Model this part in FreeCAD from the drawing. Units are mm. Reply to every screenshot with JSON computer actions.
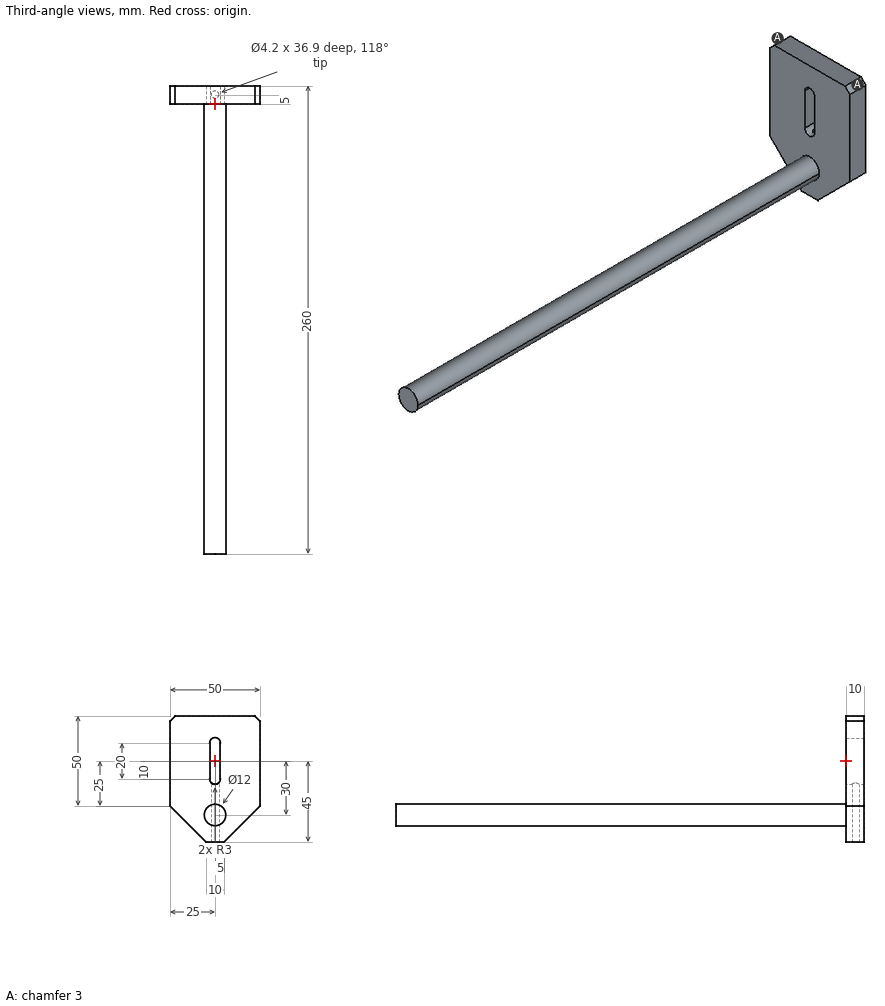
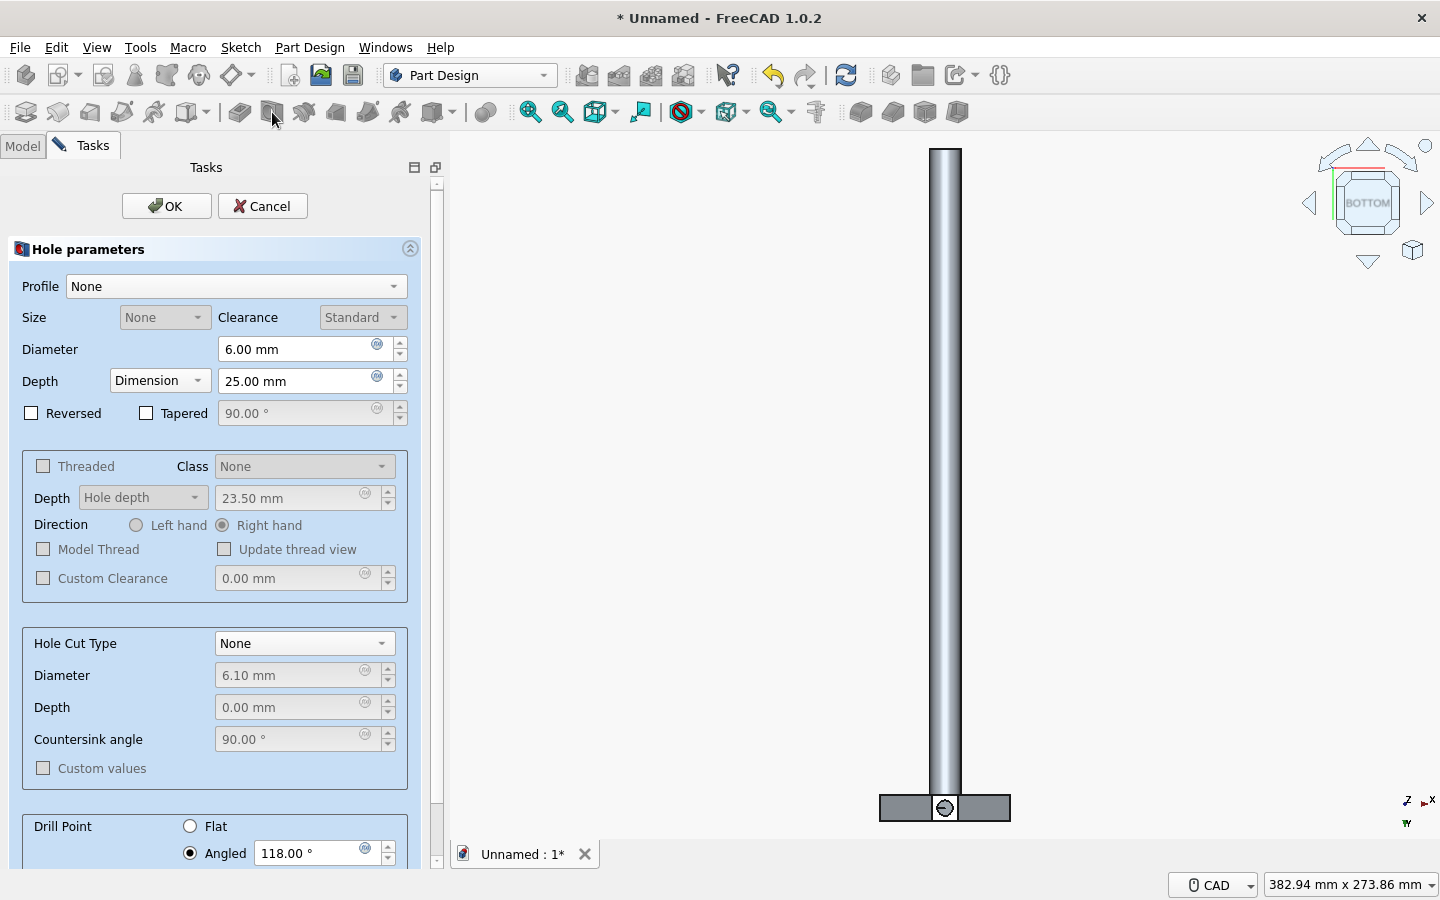
{"action": "triple_click", "coordinate": [305, 349]}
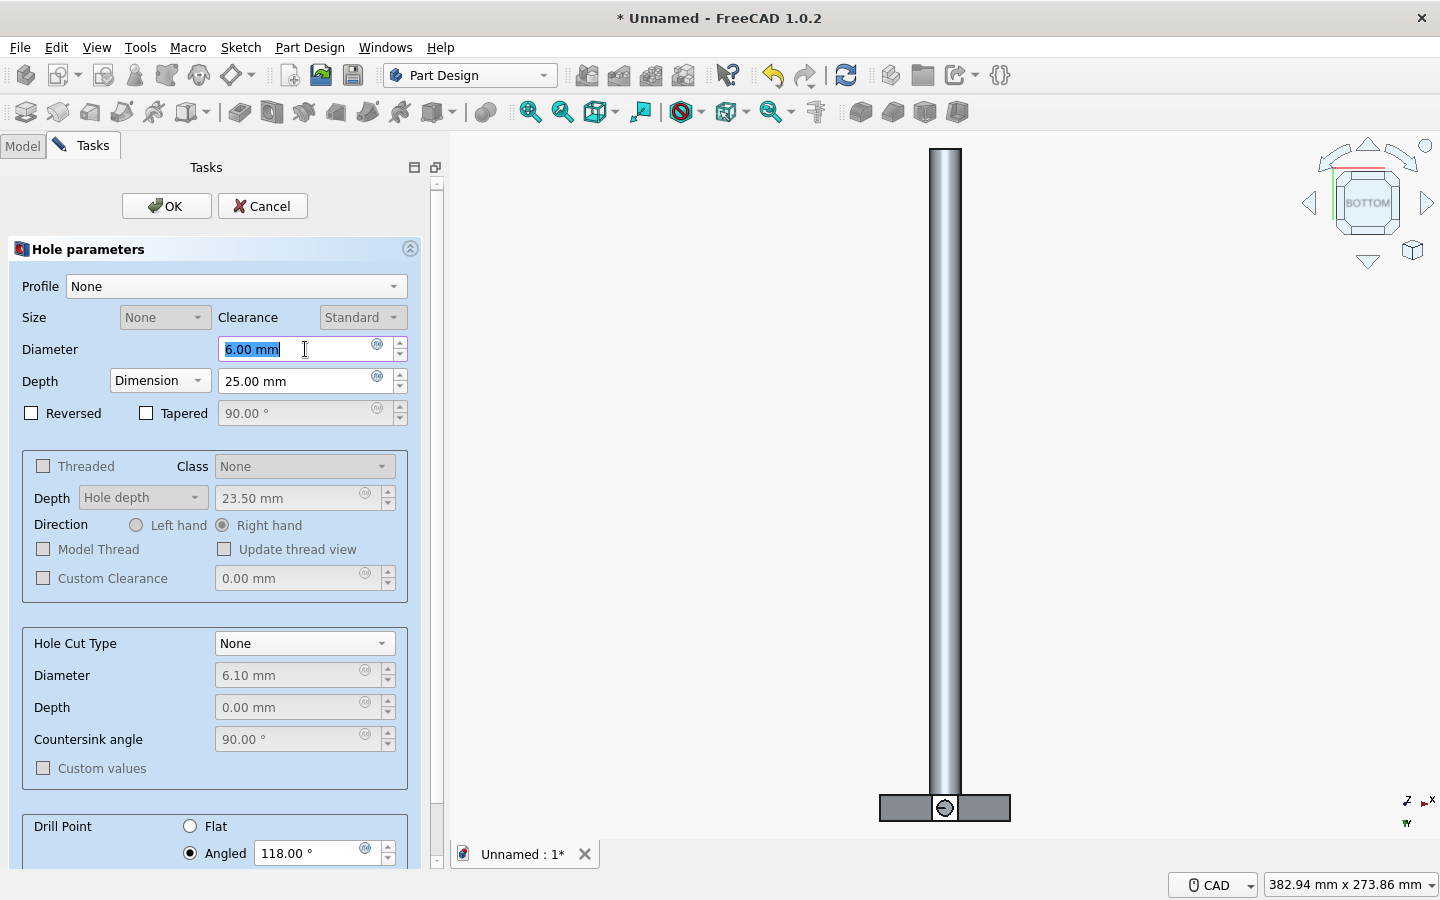
{"action": "type", "text": "4.2"}
{"action": "key", "text": "Tab"}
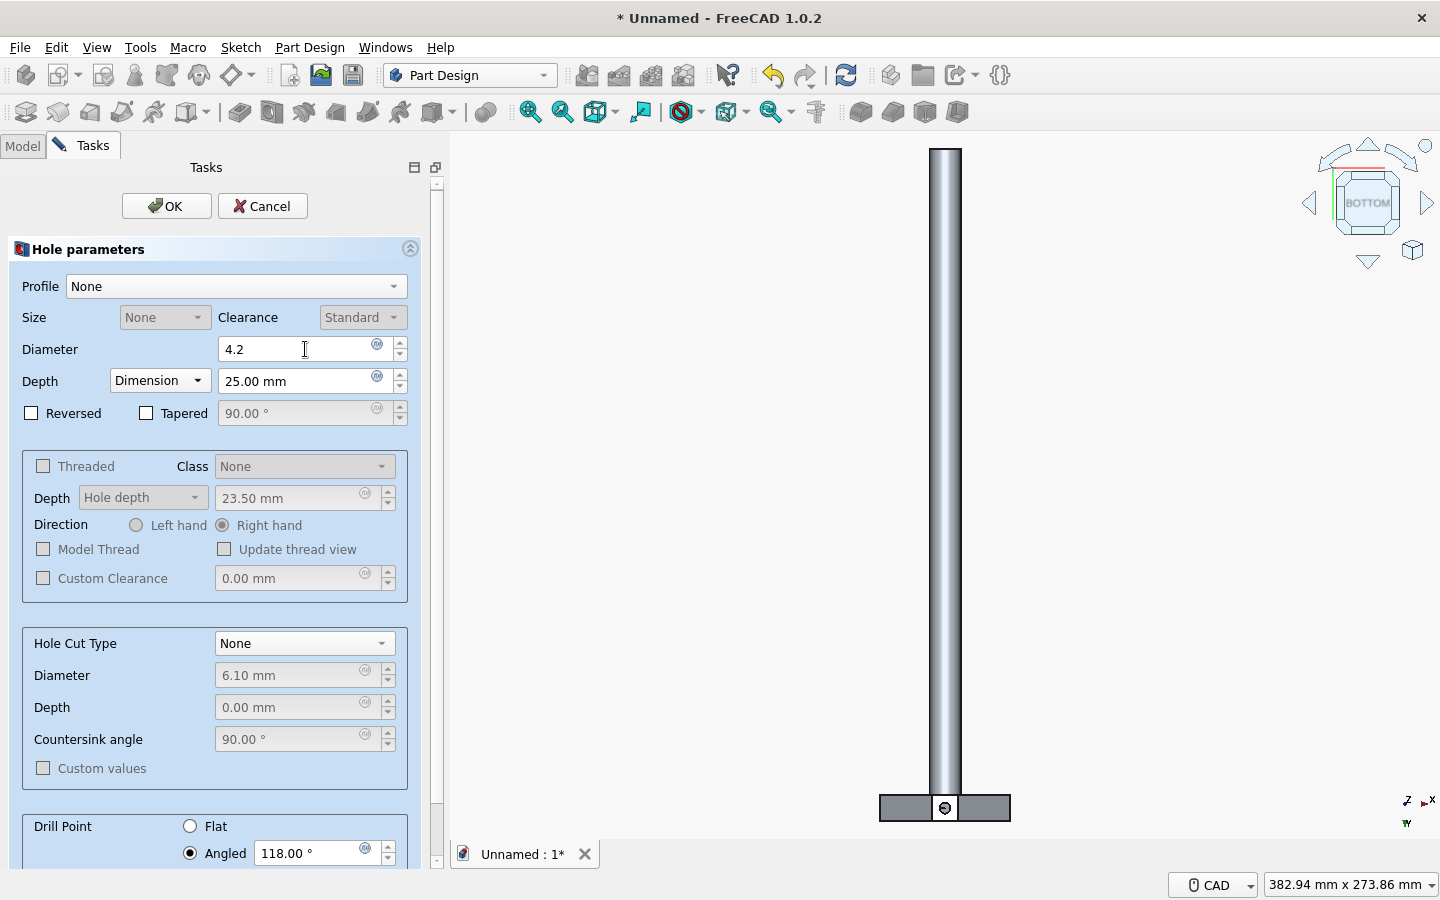
{"action": "triple_click", "coordinate": [305, 381]}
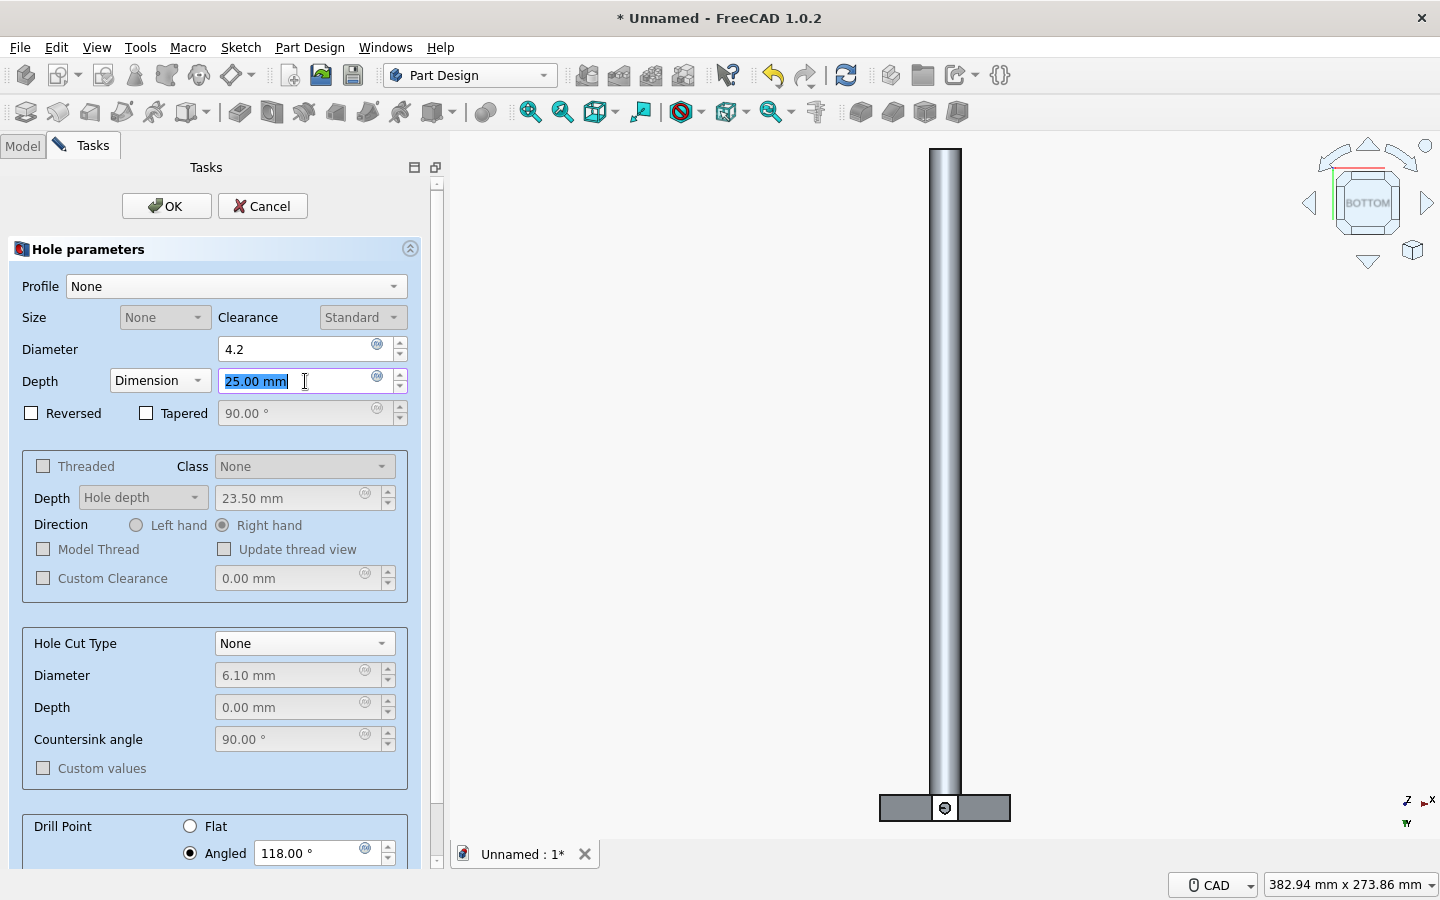
{"action": "type", "text": "36.9"}
{"action": "key", "text": "Tab"}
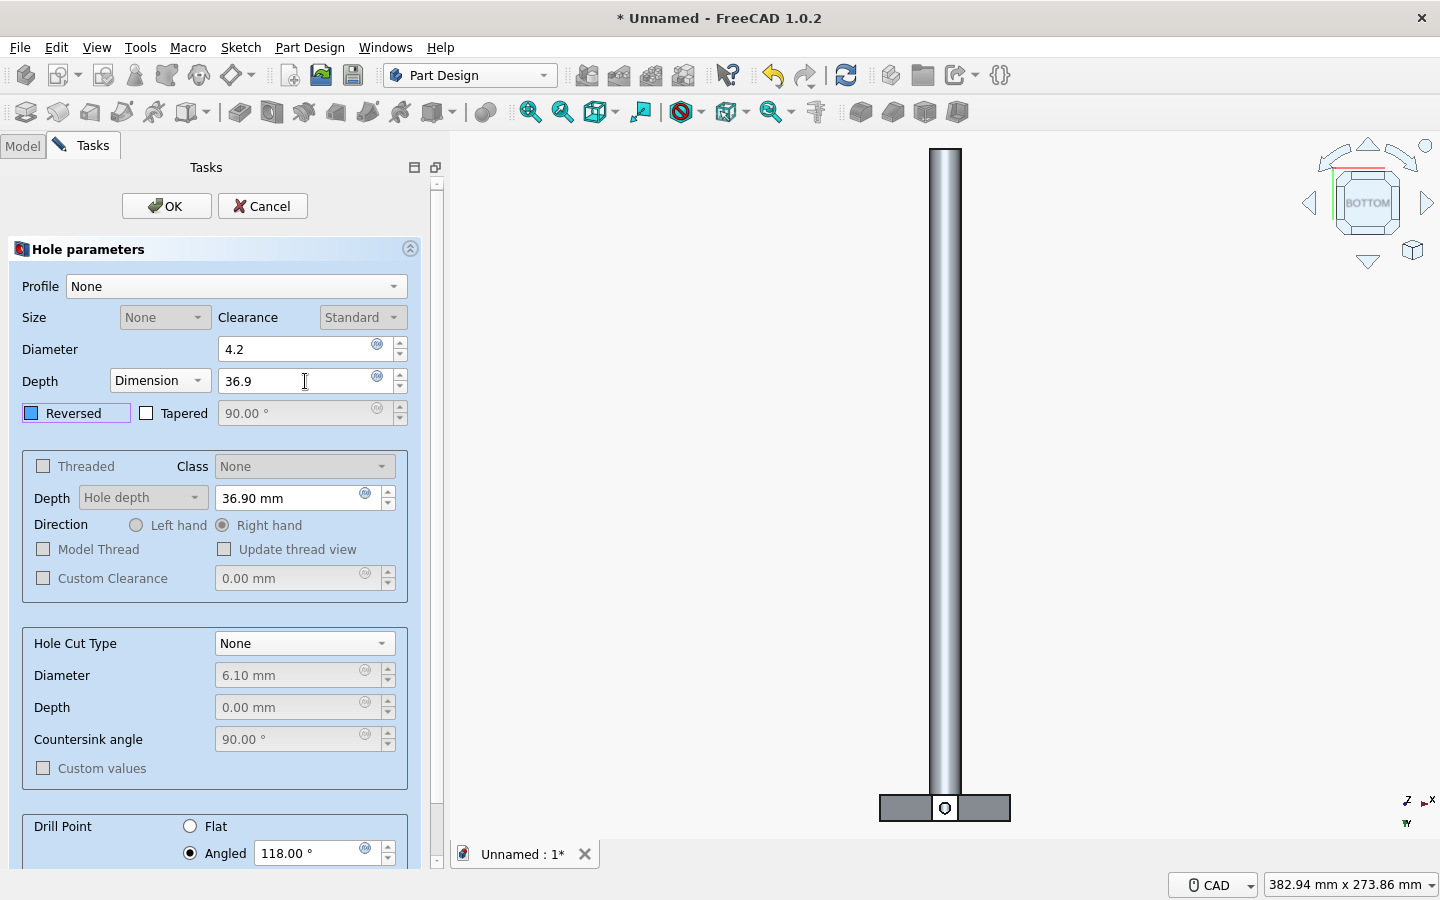
{"action": "left_click", "coordinate": [167, 206]}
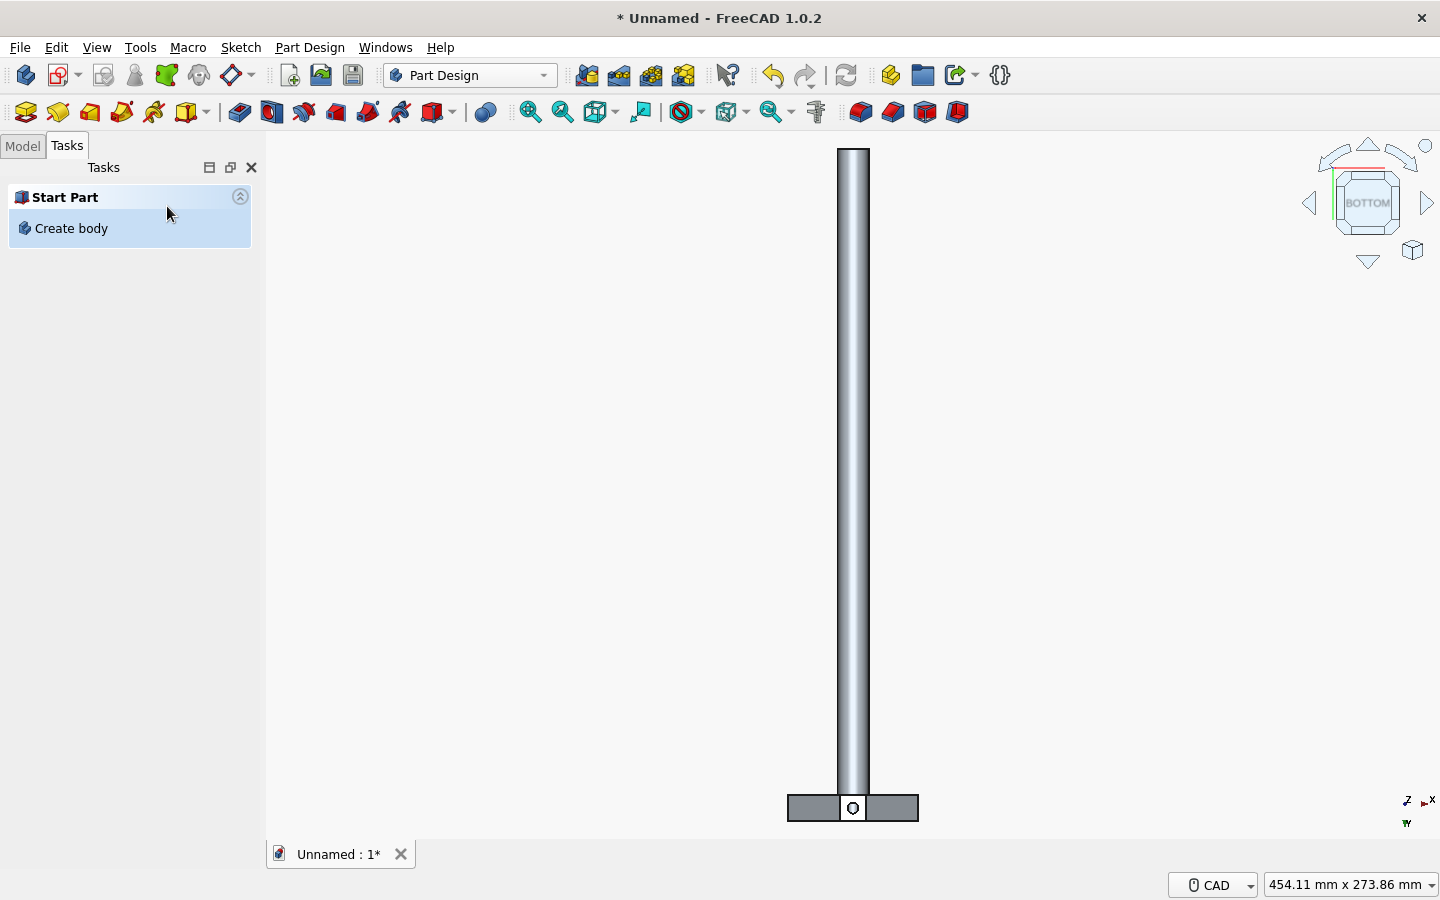
{"action": "key", "text": "0"}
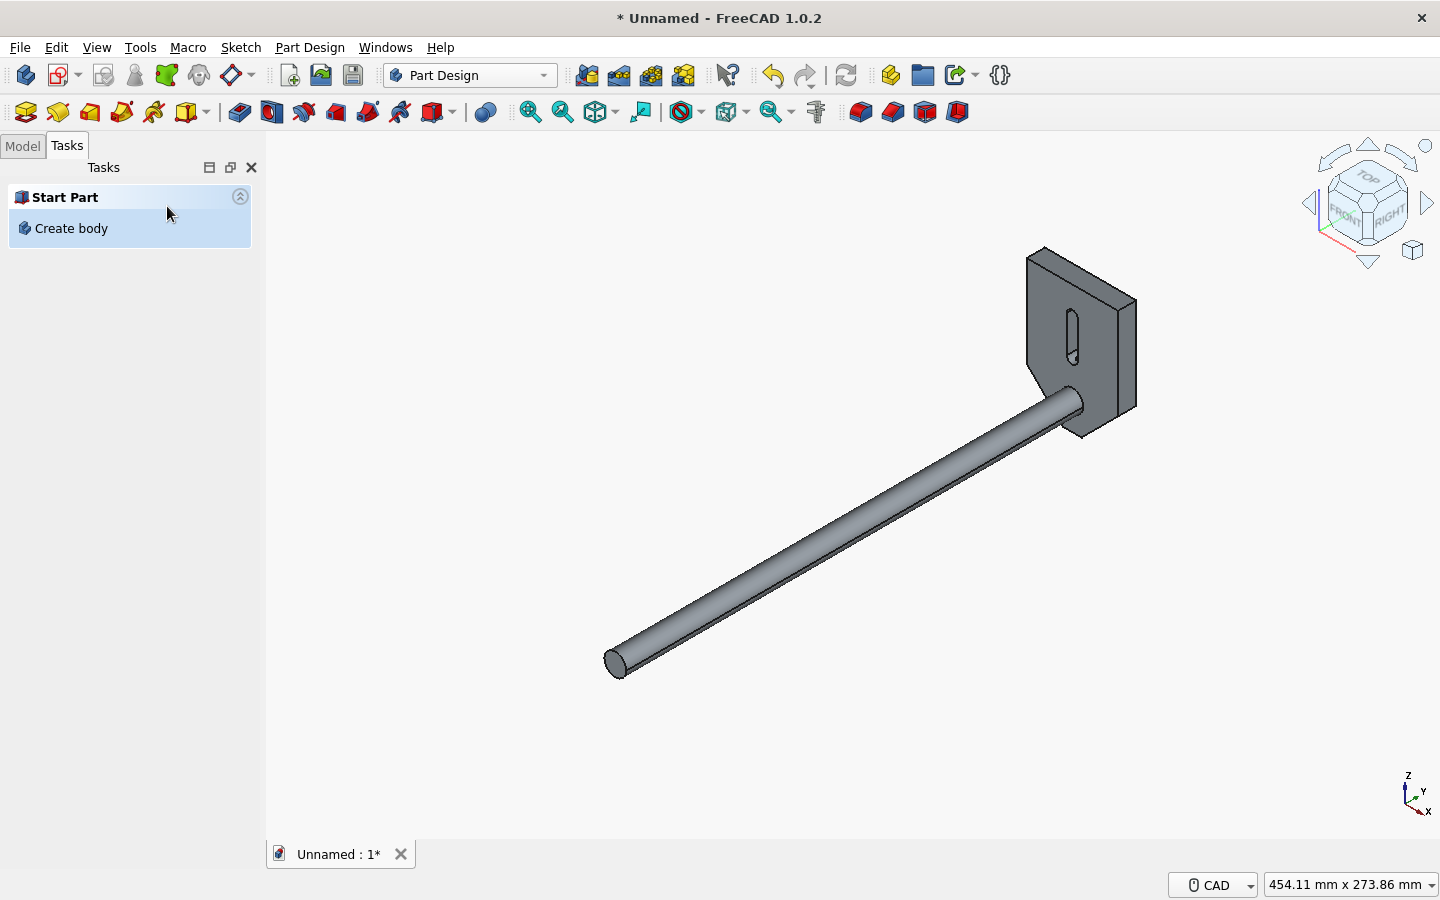
{"action": "left_click", "coordinate": [1127, 305]}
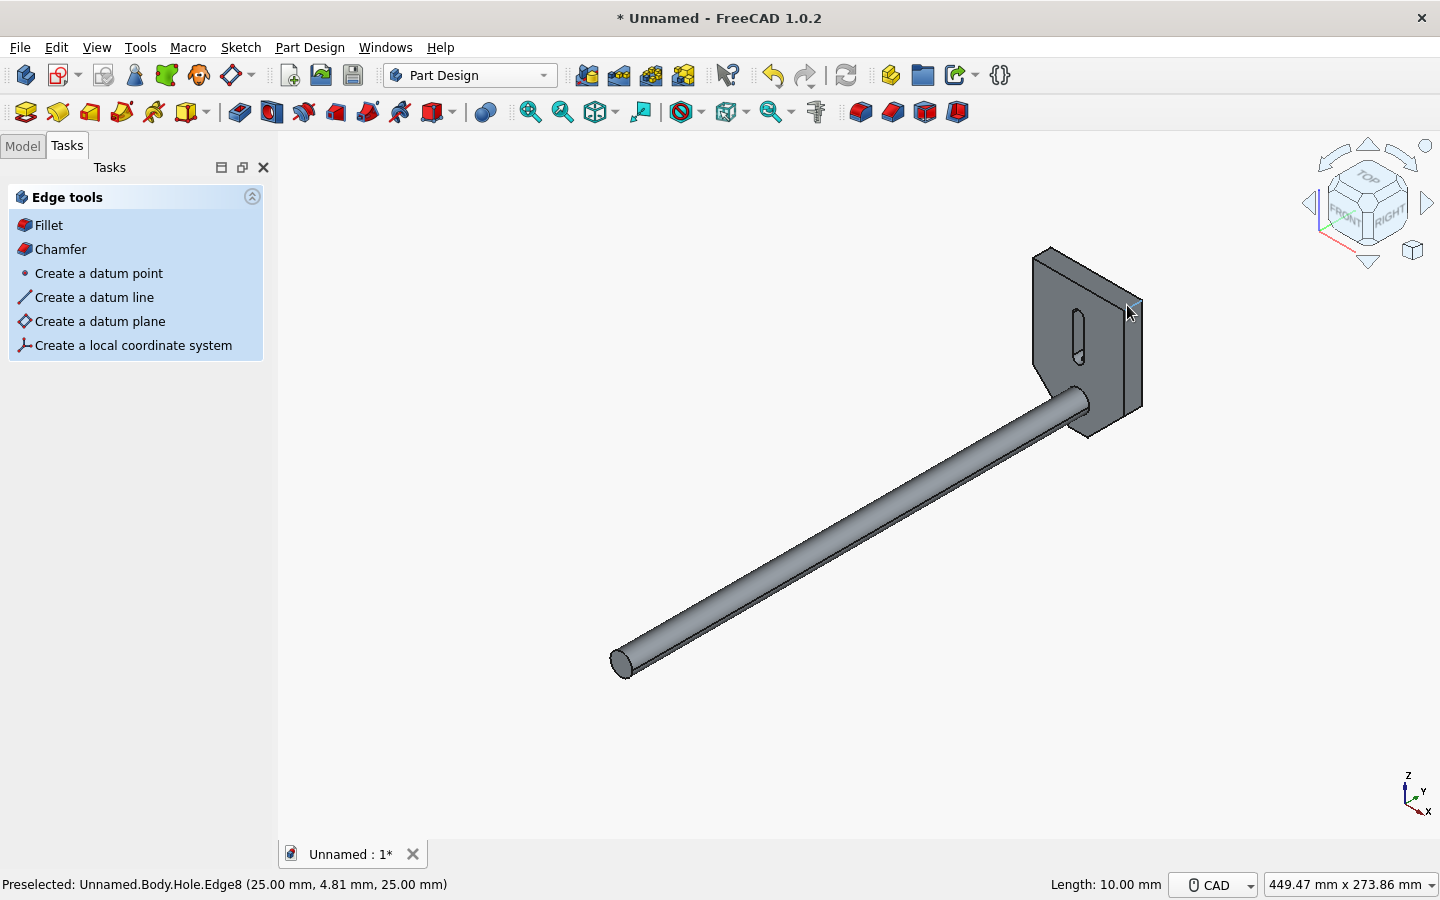
{"action": "key", "text": "2"}